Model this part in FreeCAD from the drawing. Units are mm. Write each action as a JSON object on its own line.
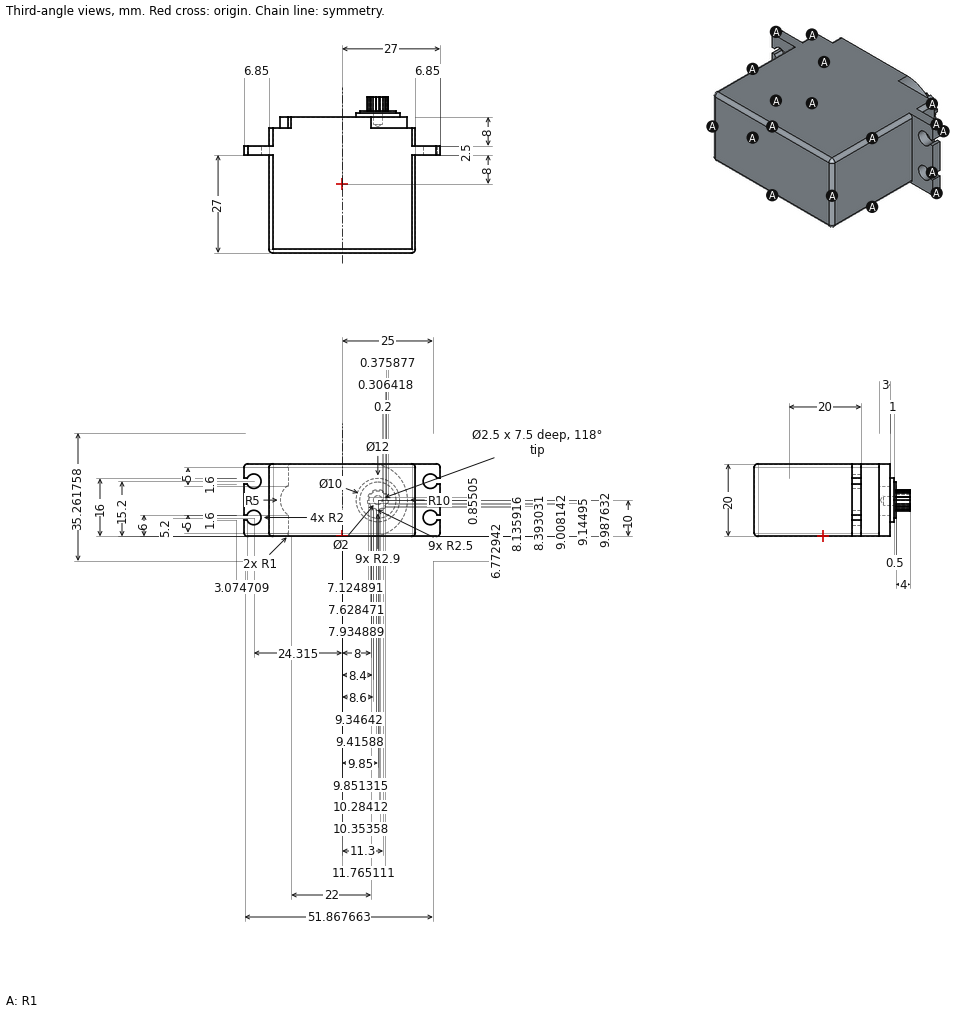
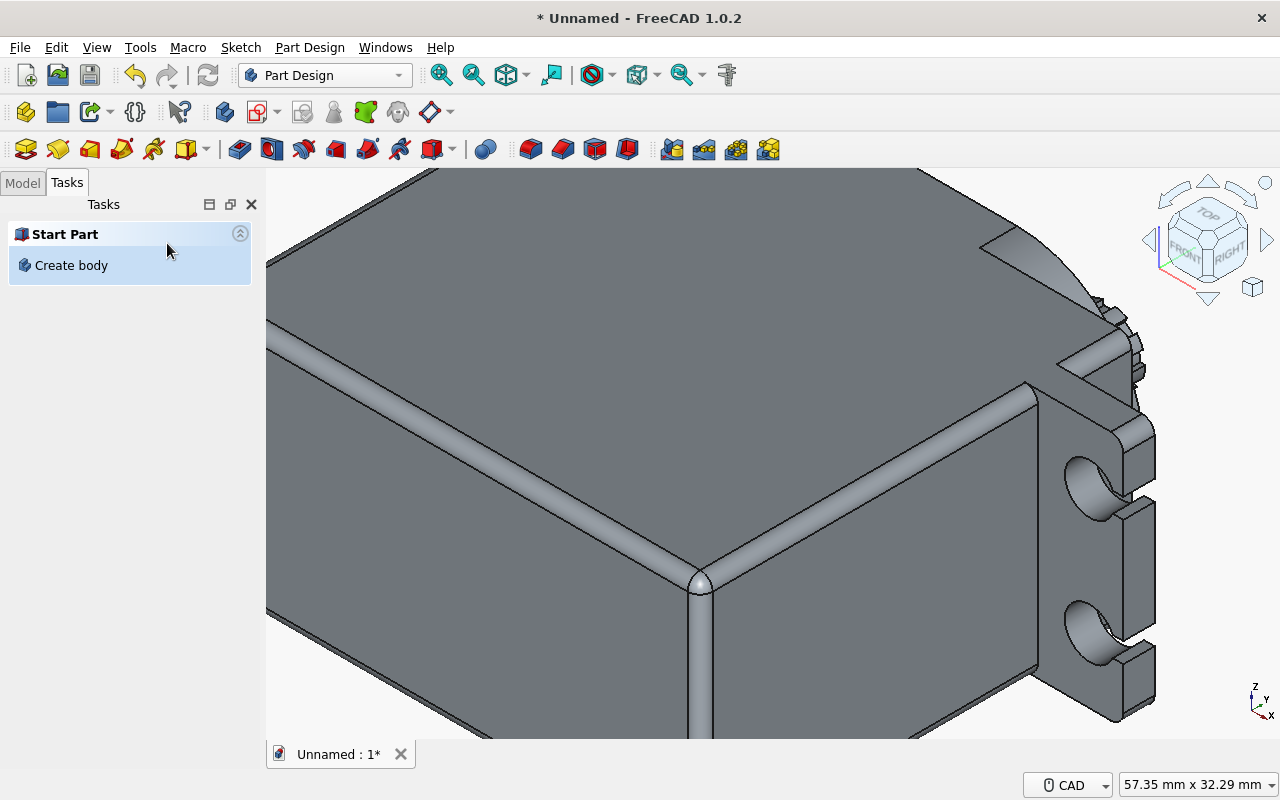
{"action": "key", "text": "v f"}